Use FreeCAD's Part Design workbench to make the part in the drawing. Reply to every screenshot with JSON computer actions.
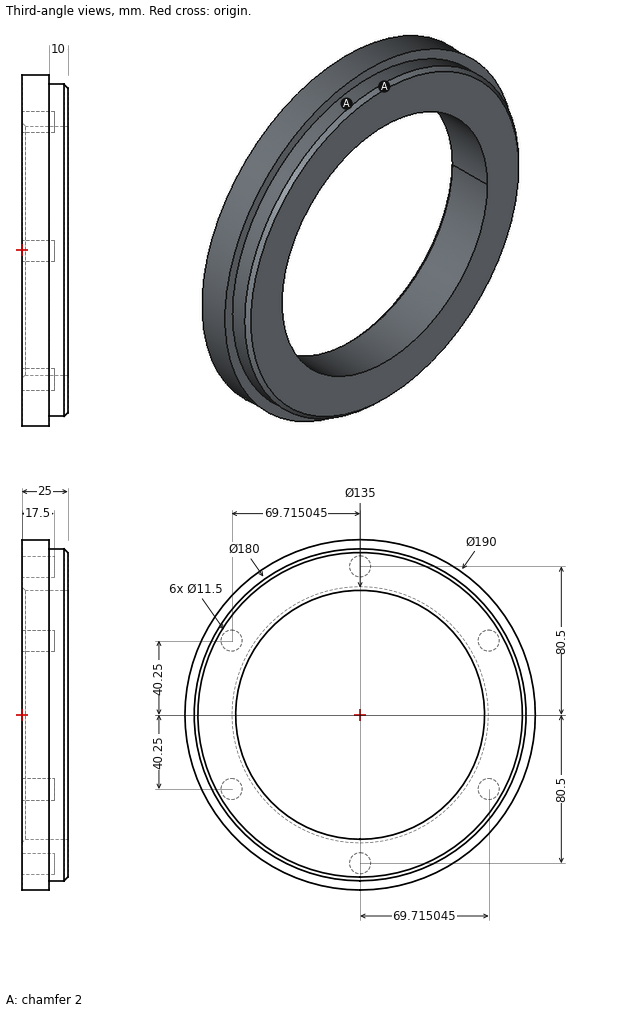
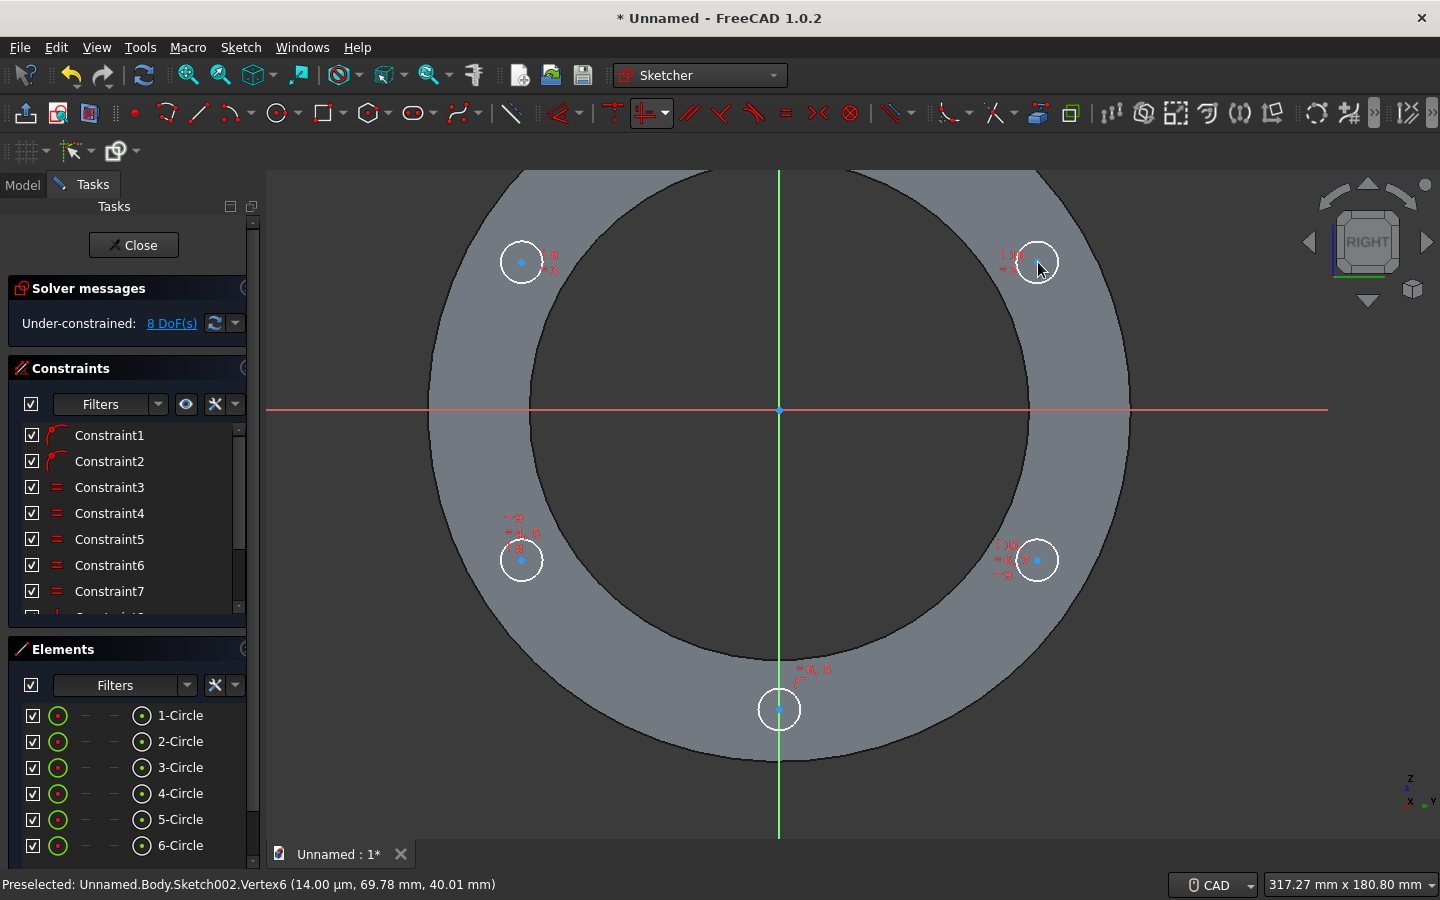
{"action": "left_click", "coordinate": [522, 262]}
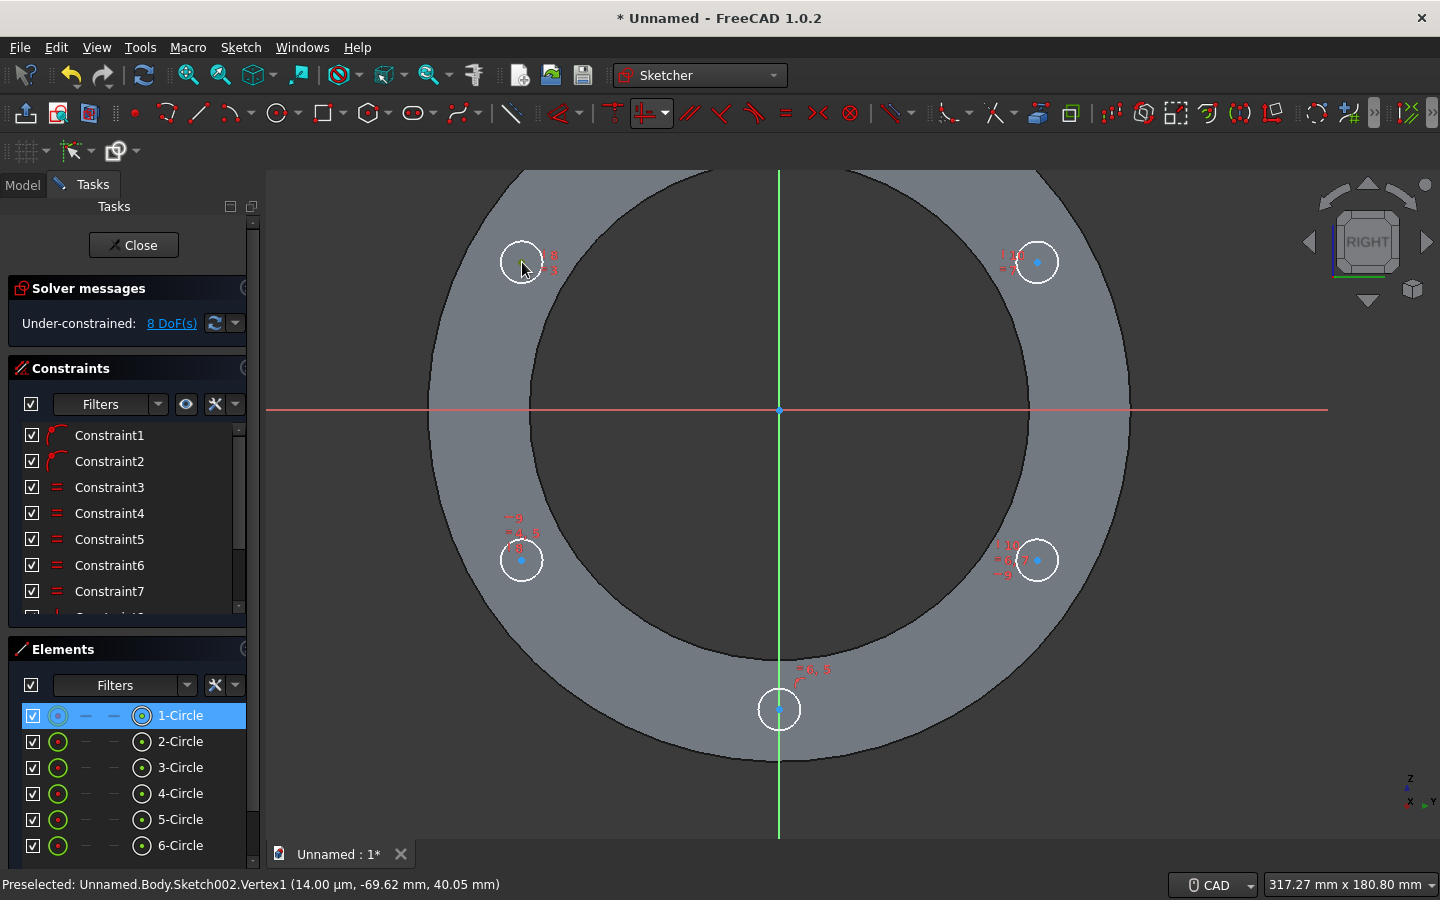
{"action": "left_click", "coordinate": [1037, 262]}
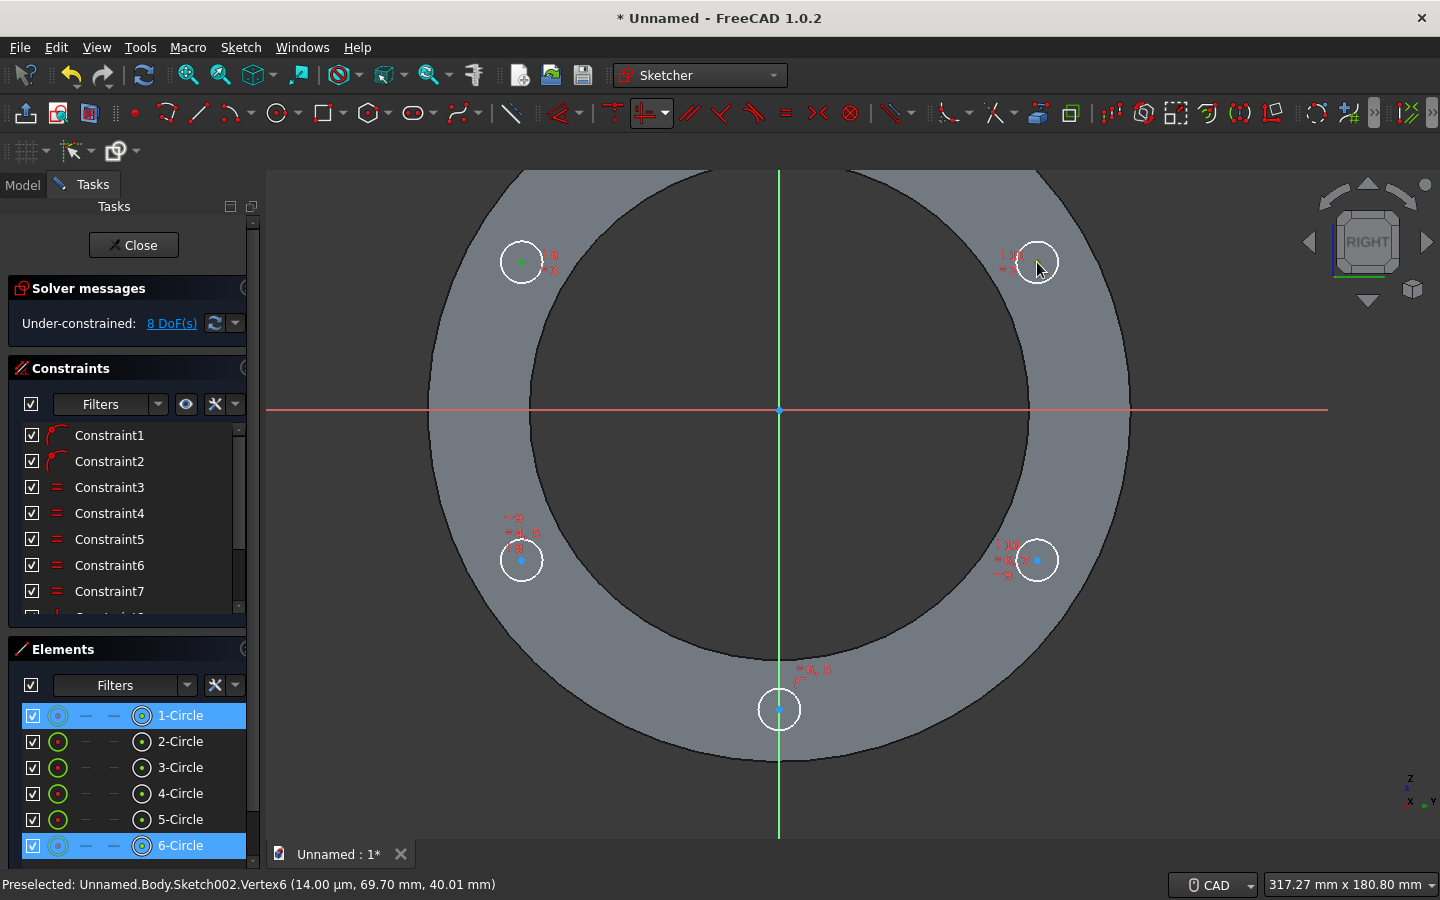
{"action": "key", "text": "h"}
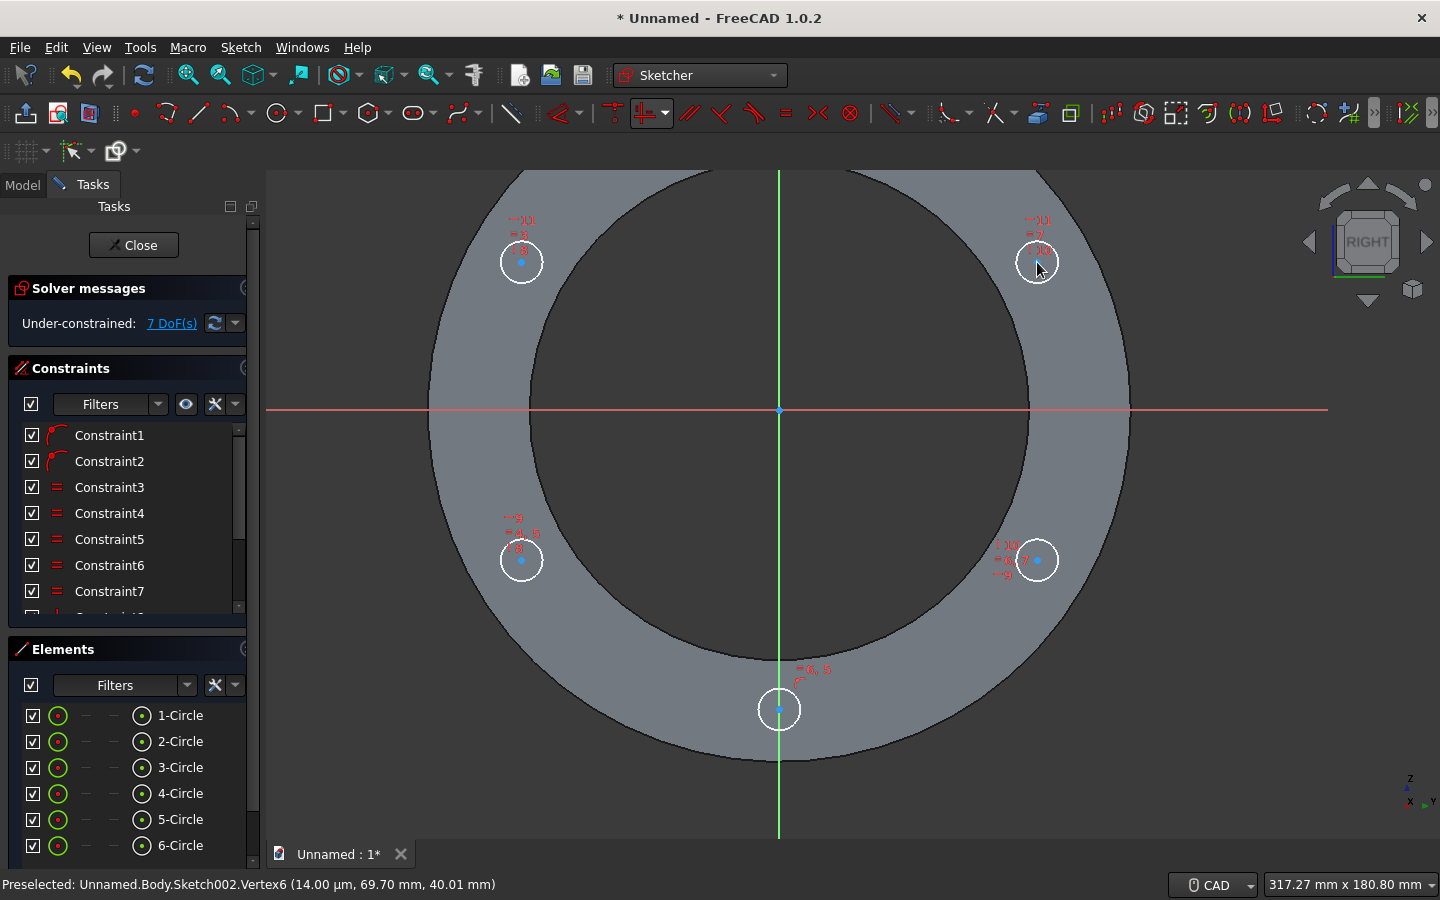
{"action": "left_click", "coordinate": [558, 114]}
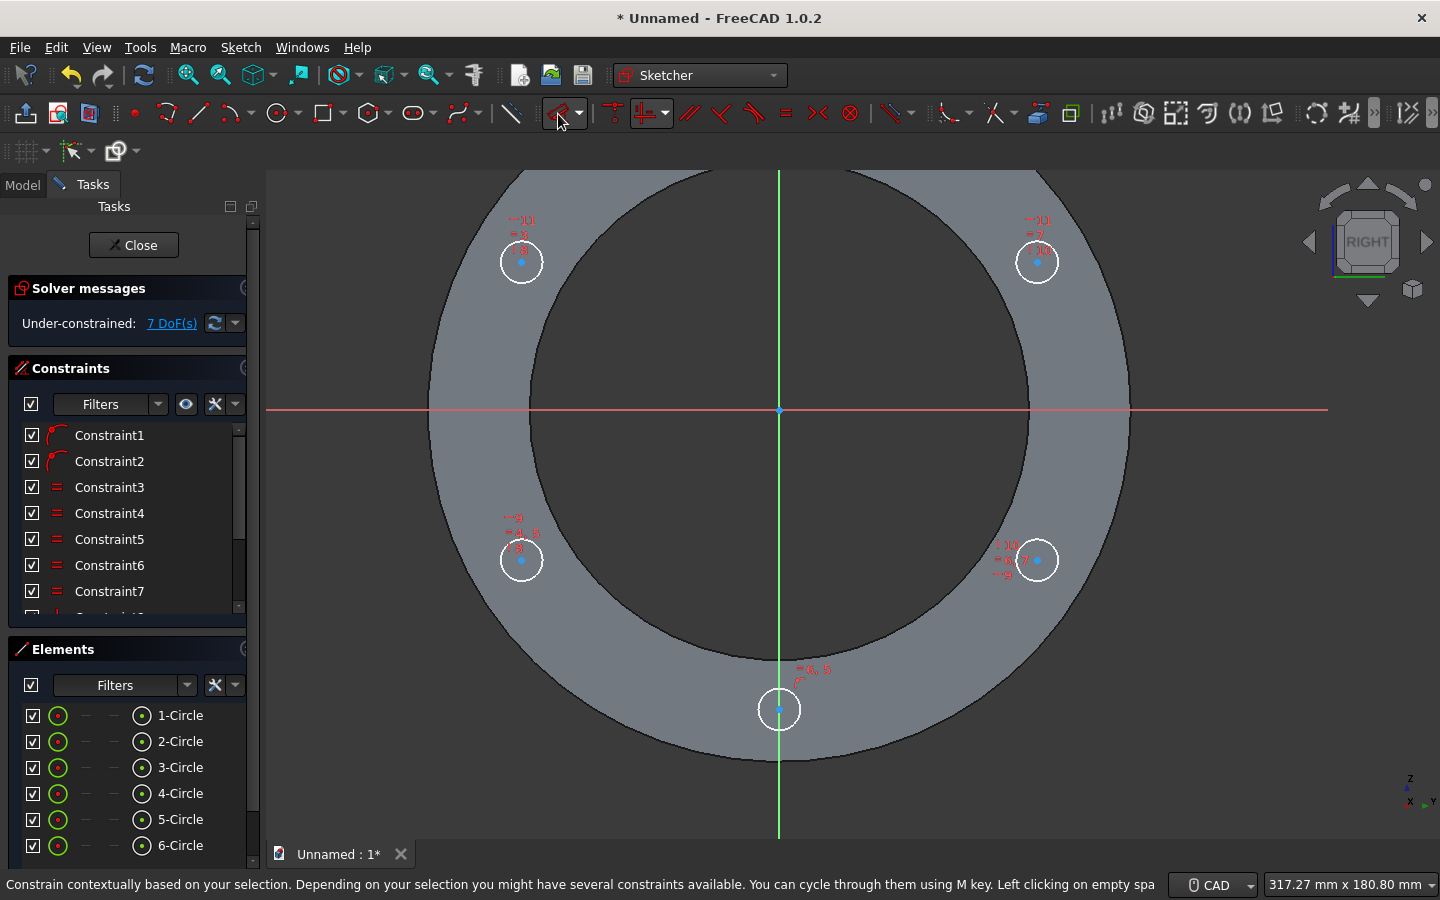
{"action": "left_click", "coordinate": [536, 247]}
{"action": "left_click", "coordinate": [558, 224]}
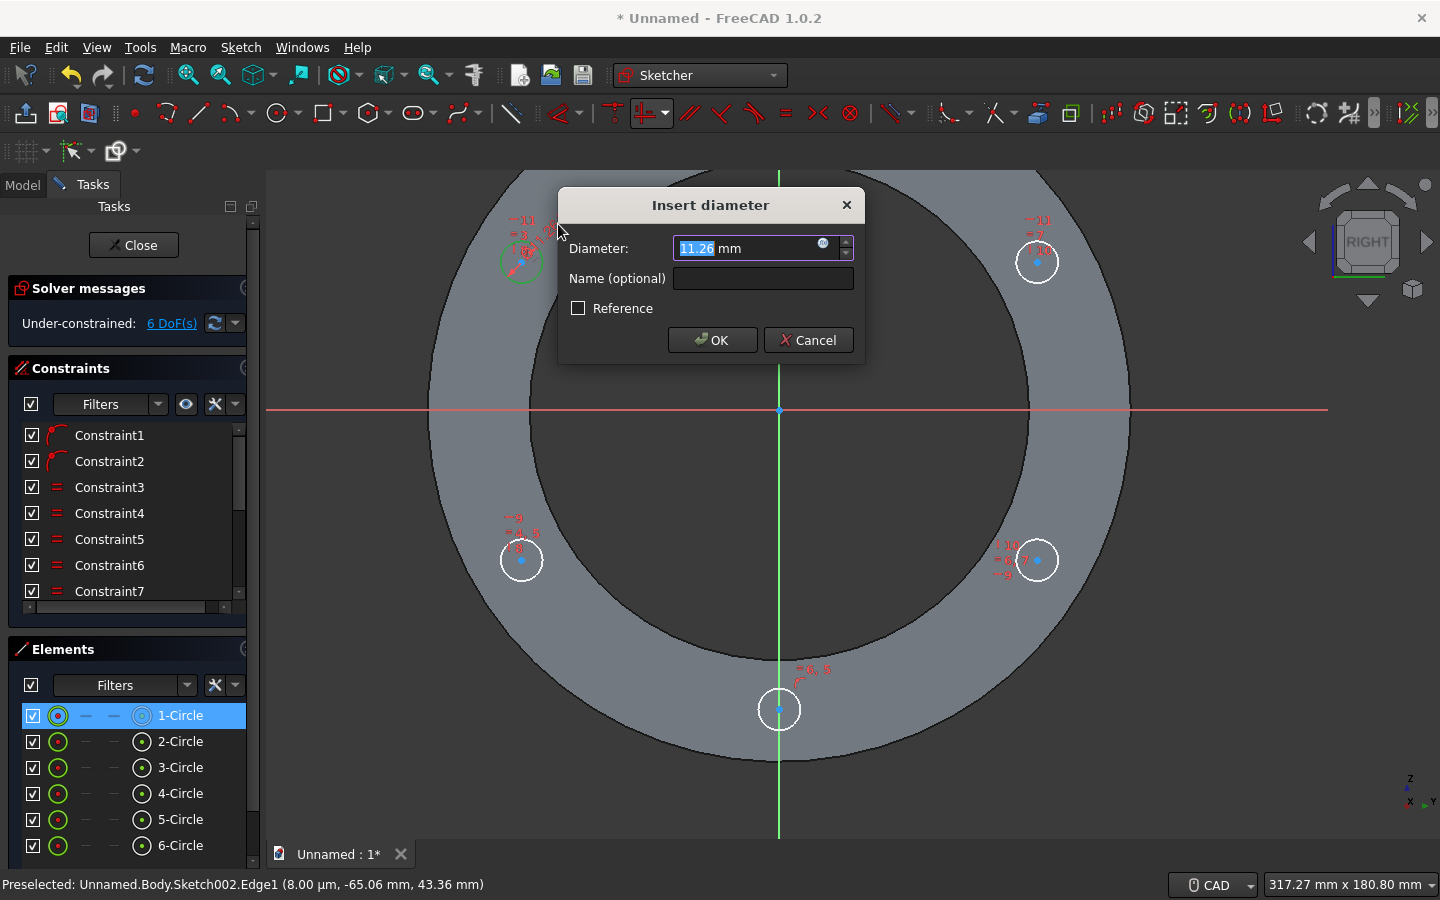
{"action": "type", "text": "11.5"}
{"action": "key", "text": "Return"}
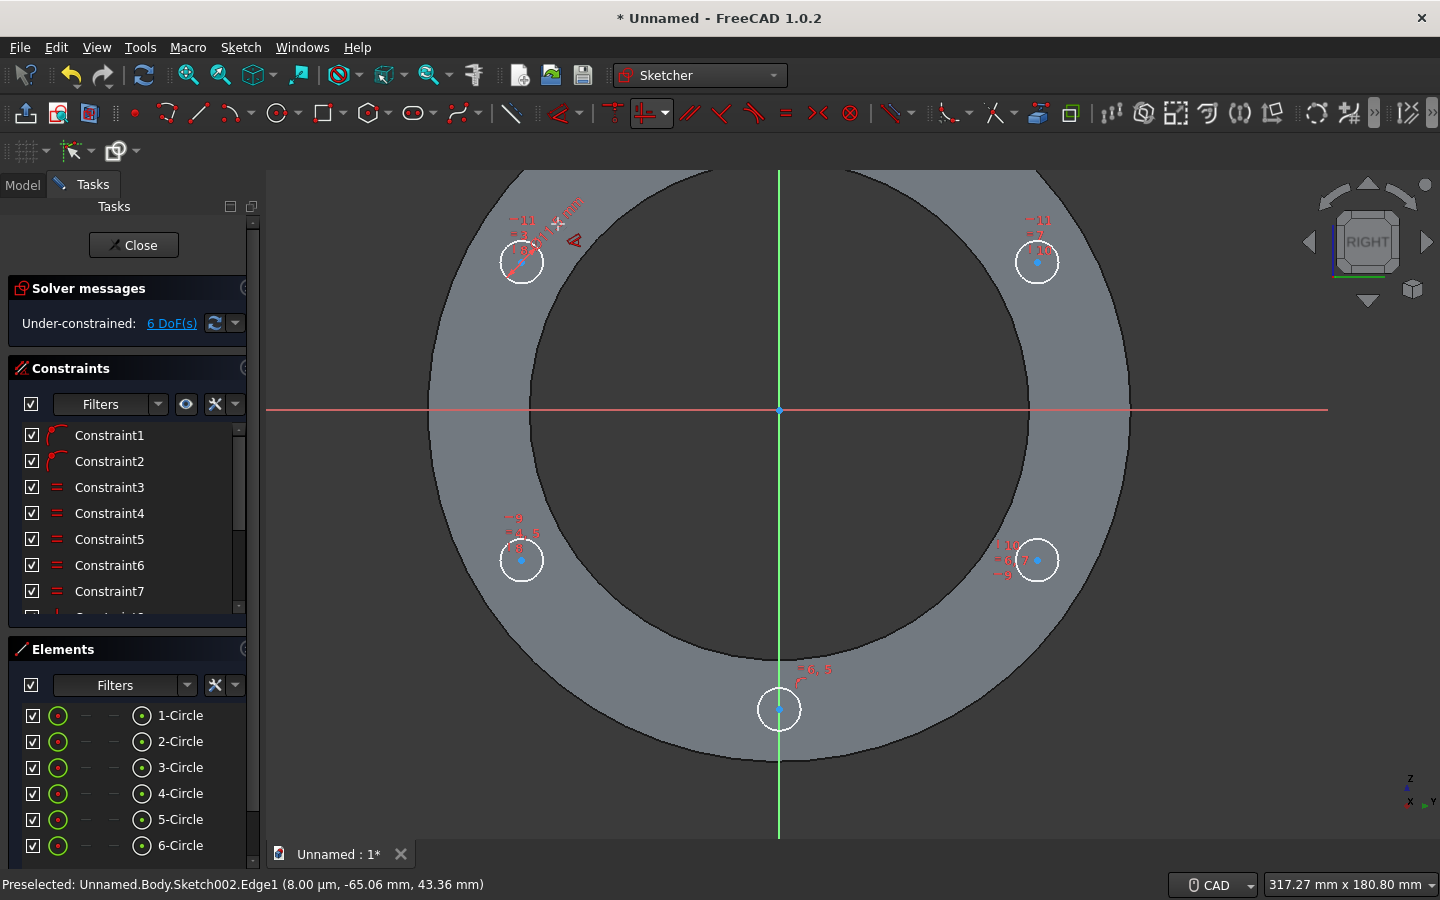
{"action": "scroll", "coordinate": [795, 696], "scroll_direction": "down", "scroll_amount": 2}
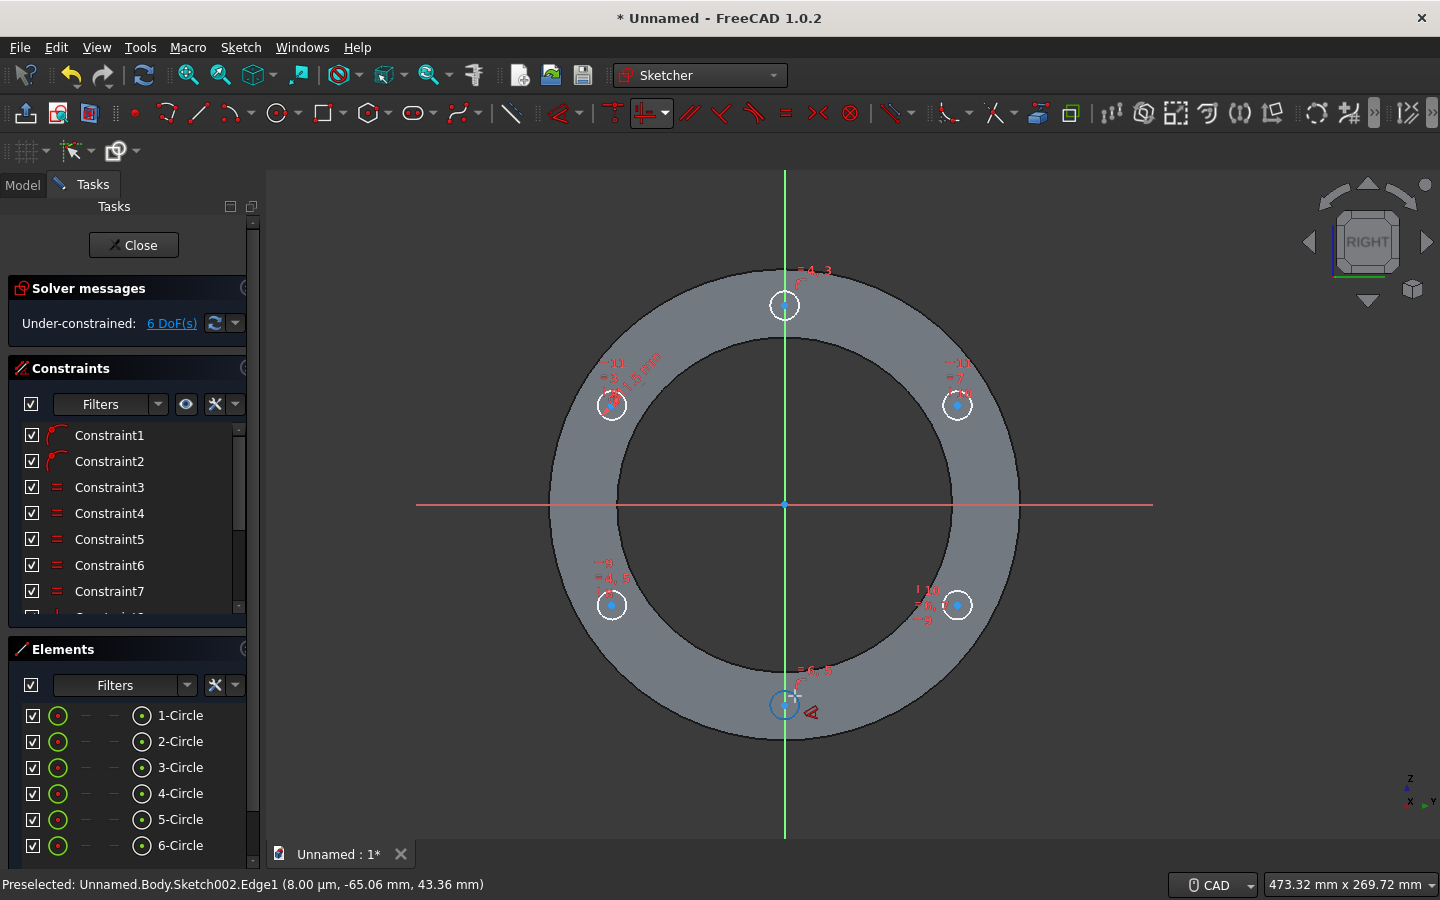
{"action": "left_click", "coordinate": [785, 306]}
{"action": "left_click", "coordinate": [819, 405]}